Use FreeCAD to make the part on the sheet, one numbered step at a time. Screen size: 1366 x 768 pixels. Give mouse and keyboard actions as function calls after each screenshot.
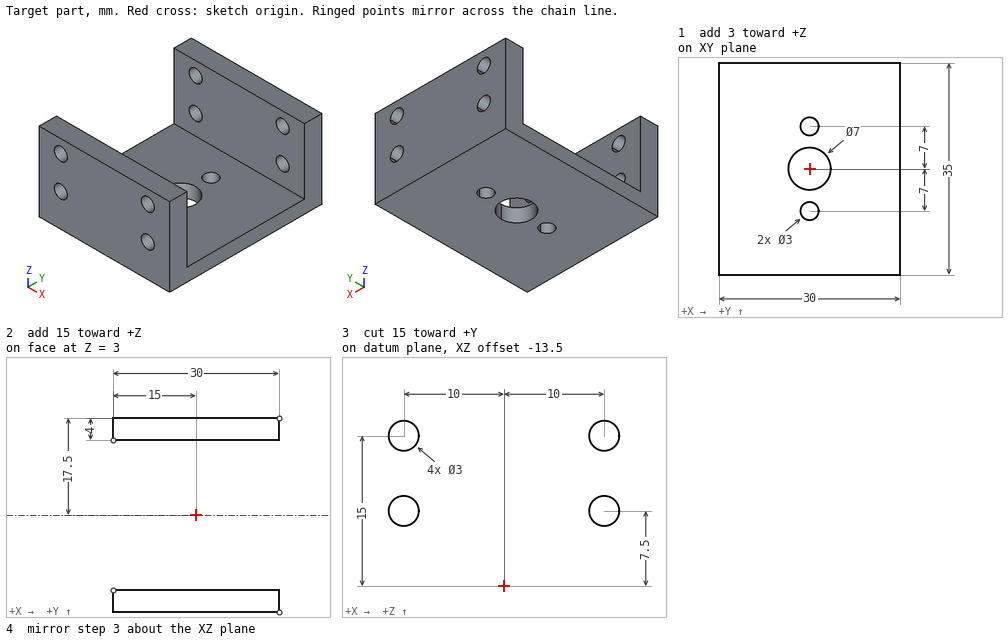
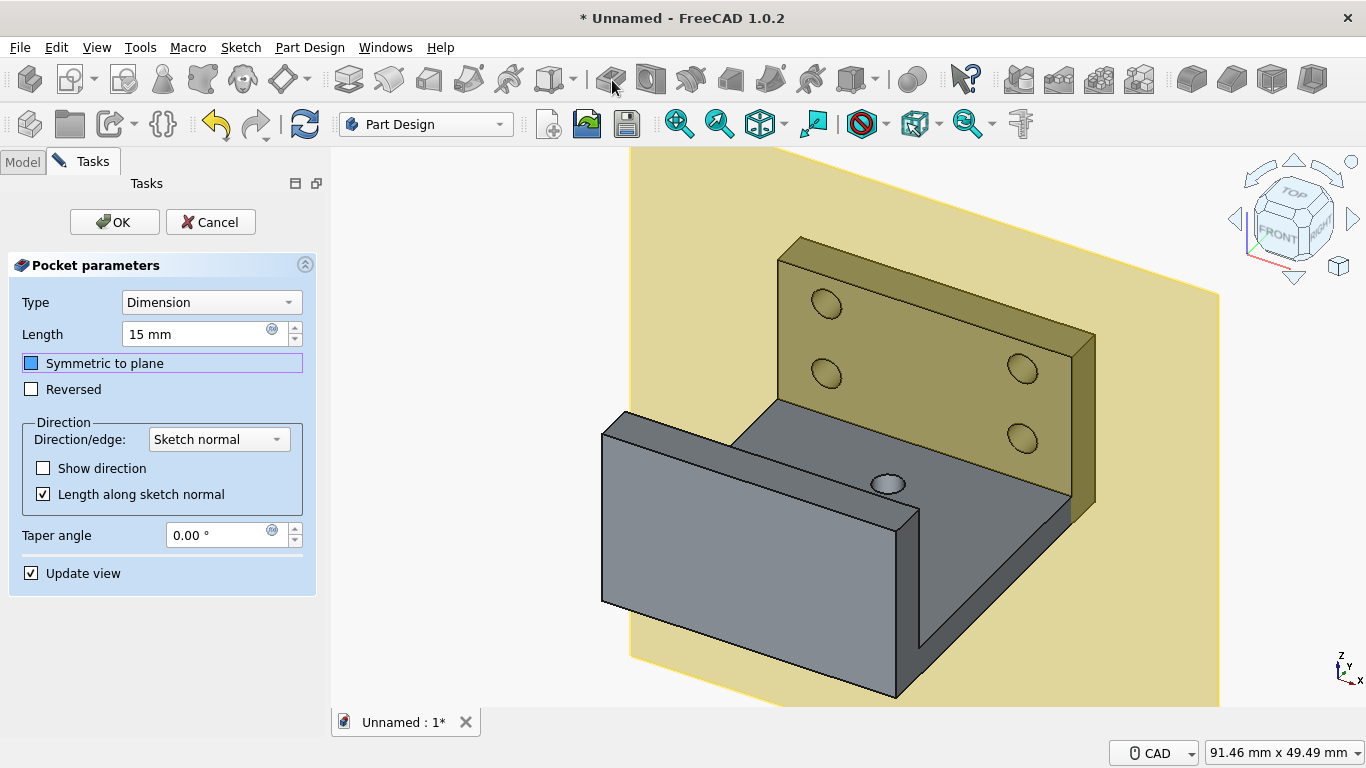
click(115, 222)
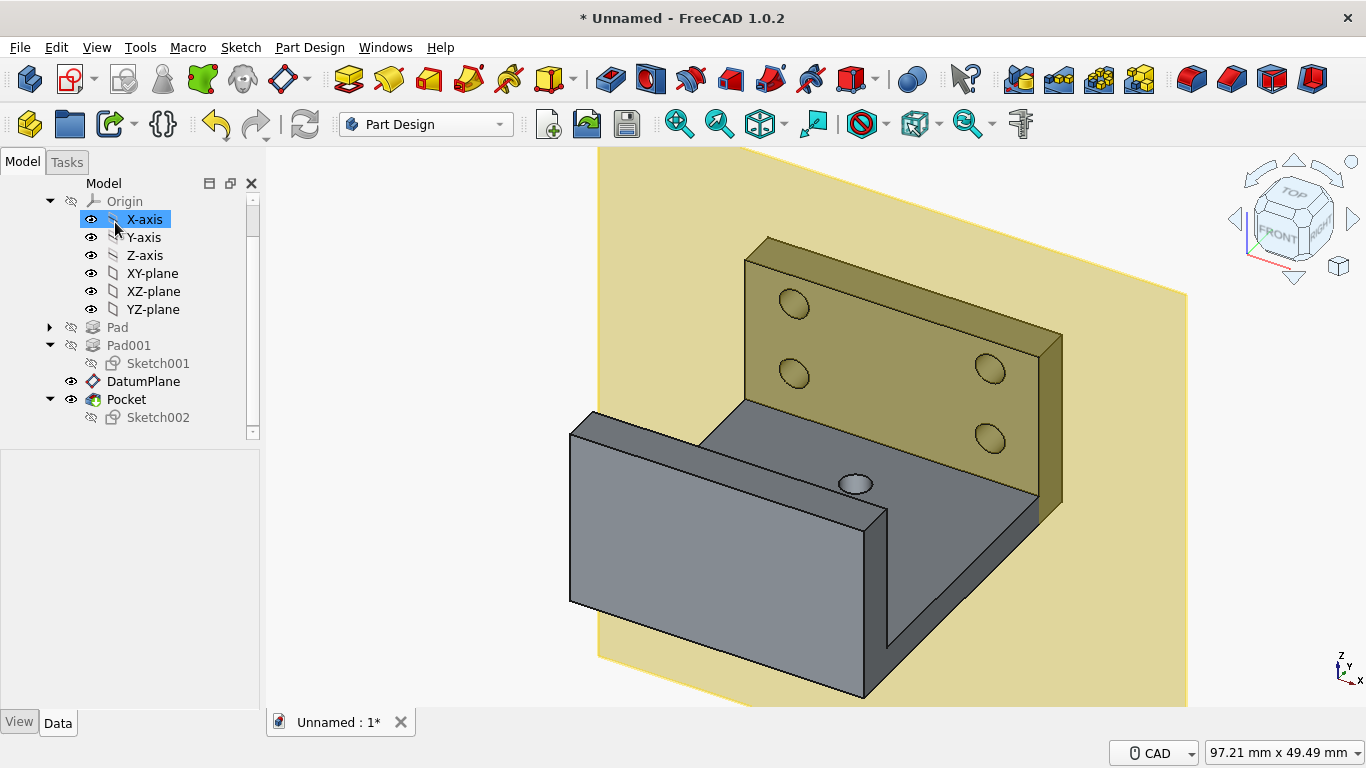
click(116, 381)
key(space)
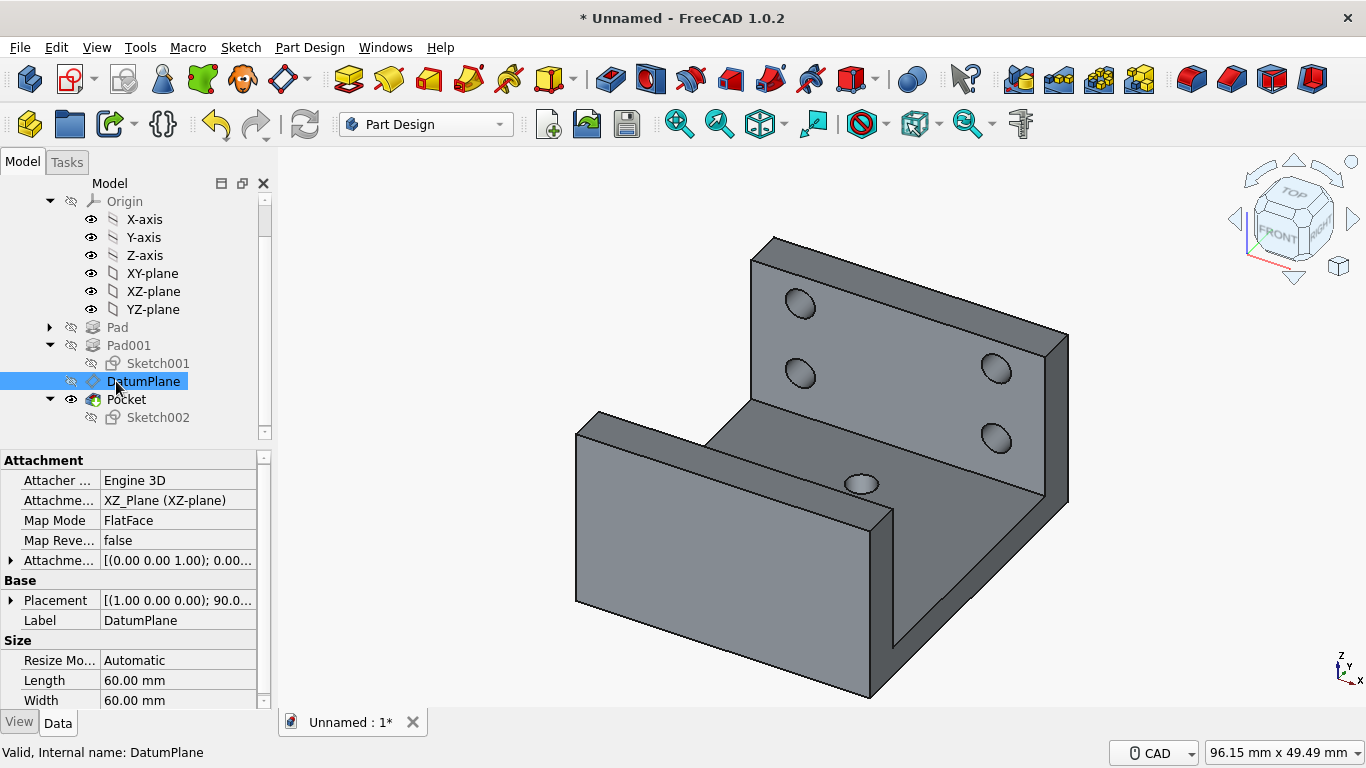
click(116, 399)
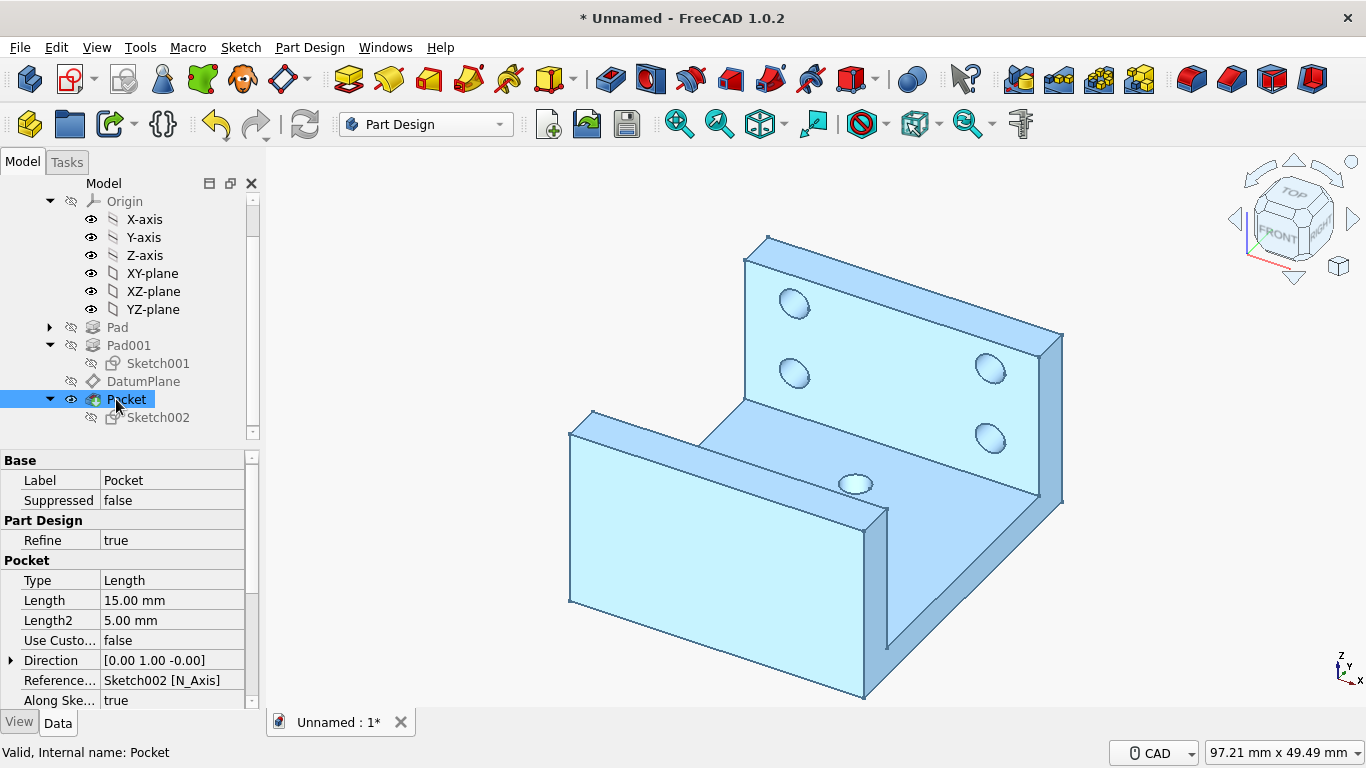
click(1020, 80)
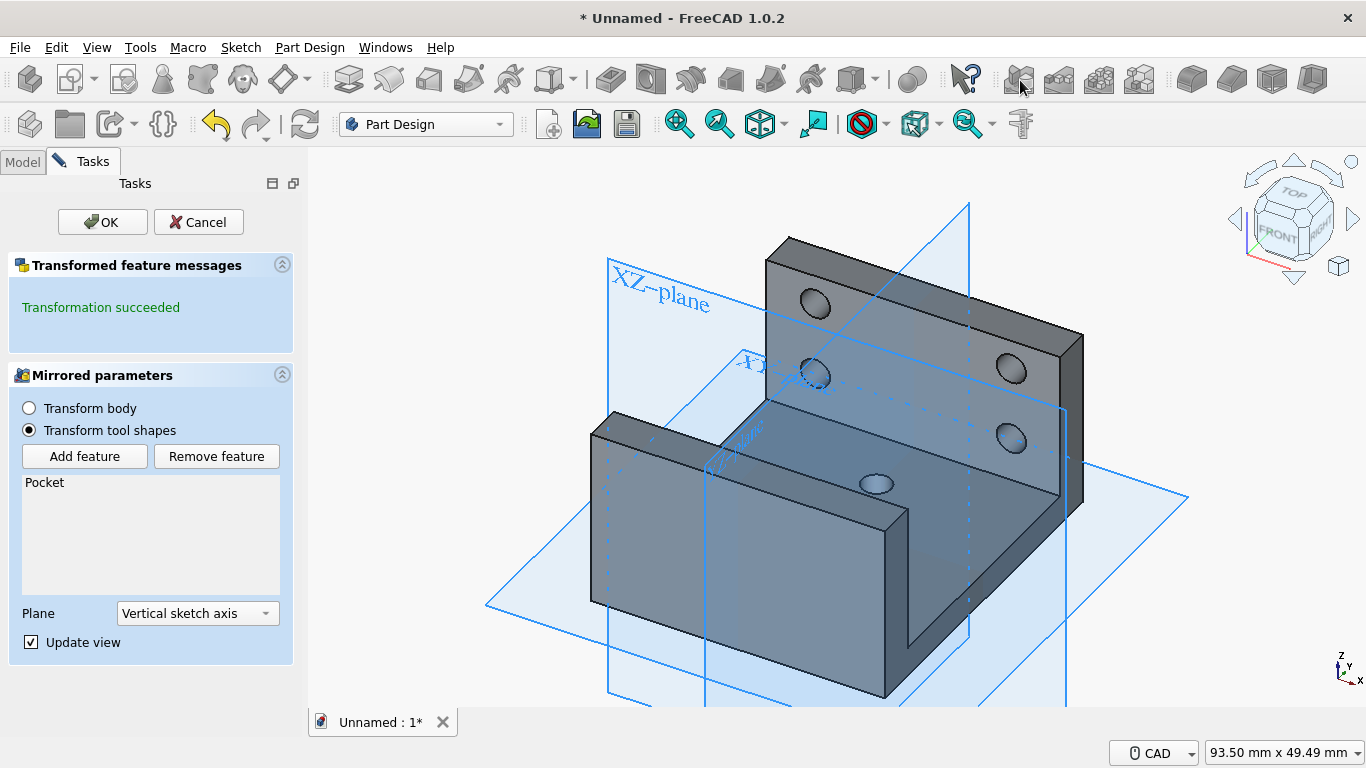
click(198, 614)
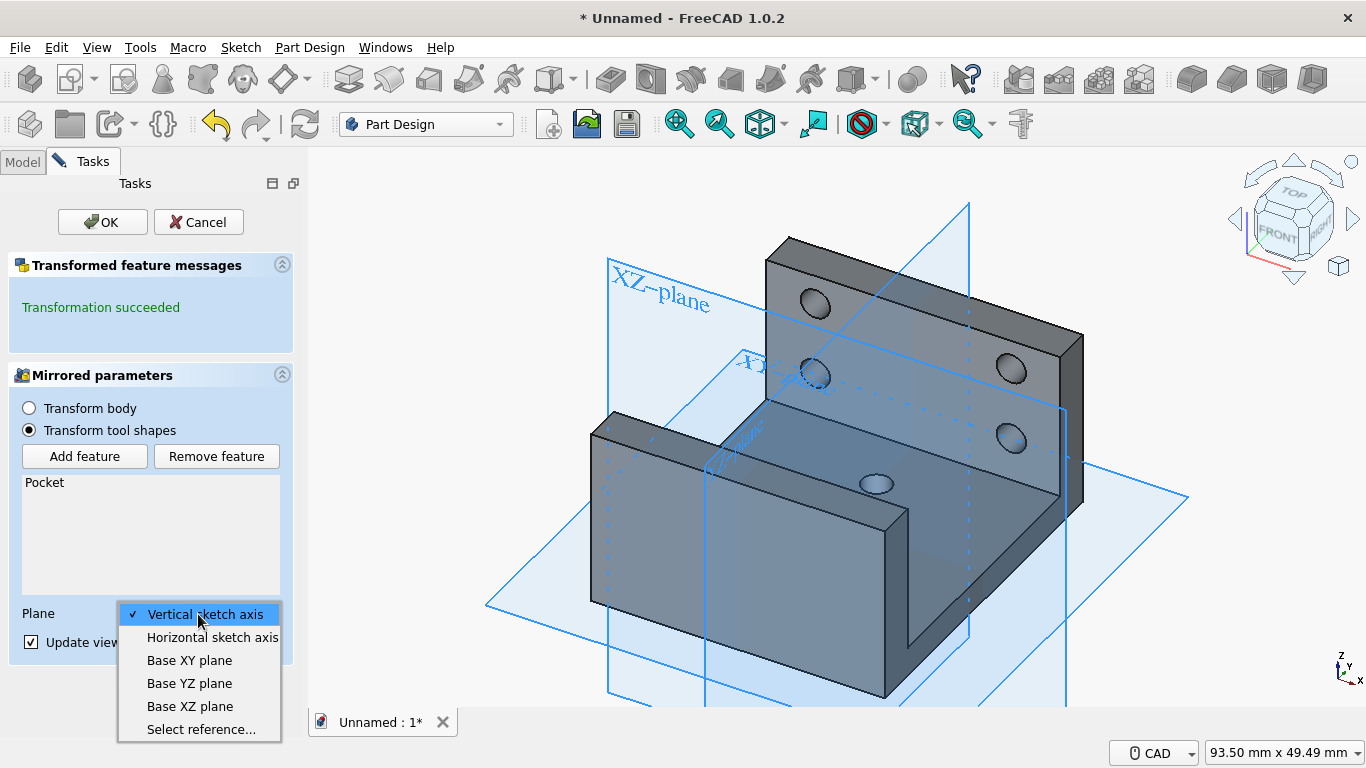
click(198, 706)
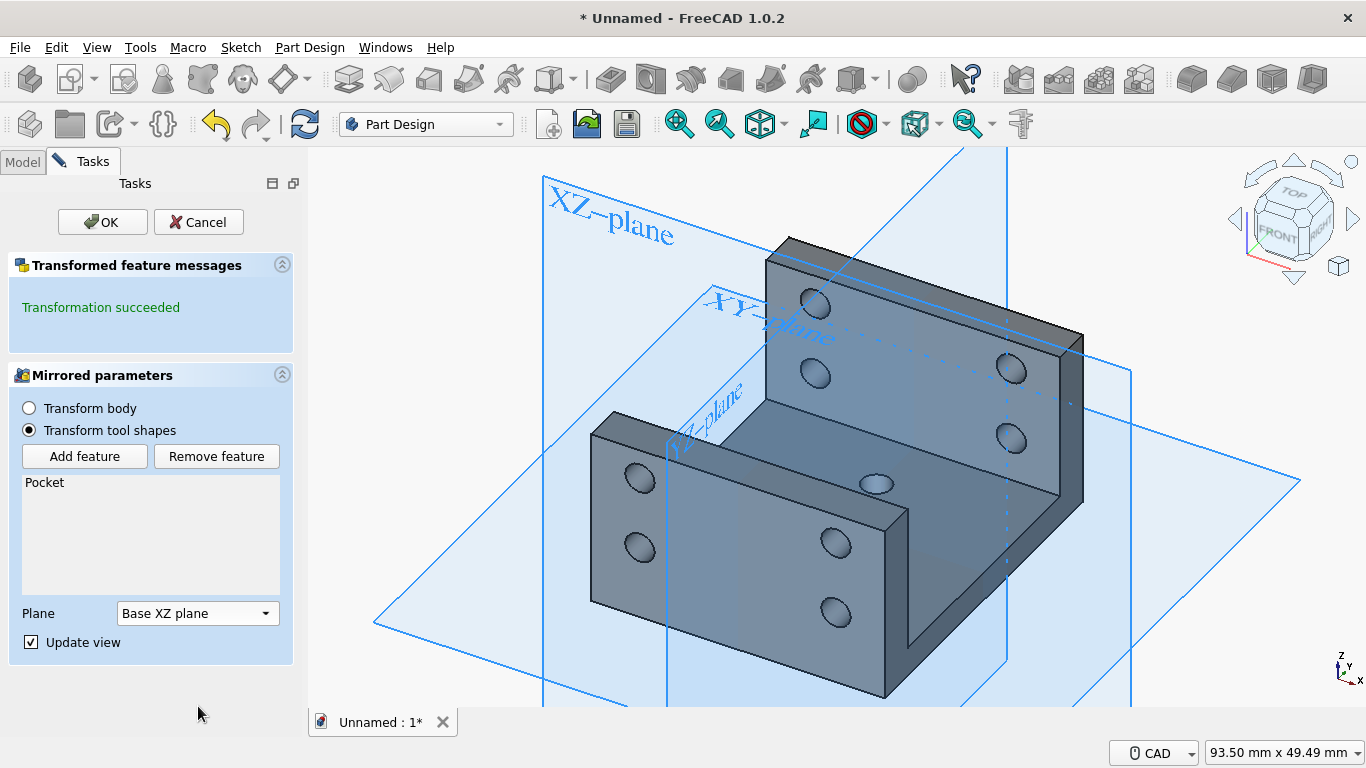
click(103, 222)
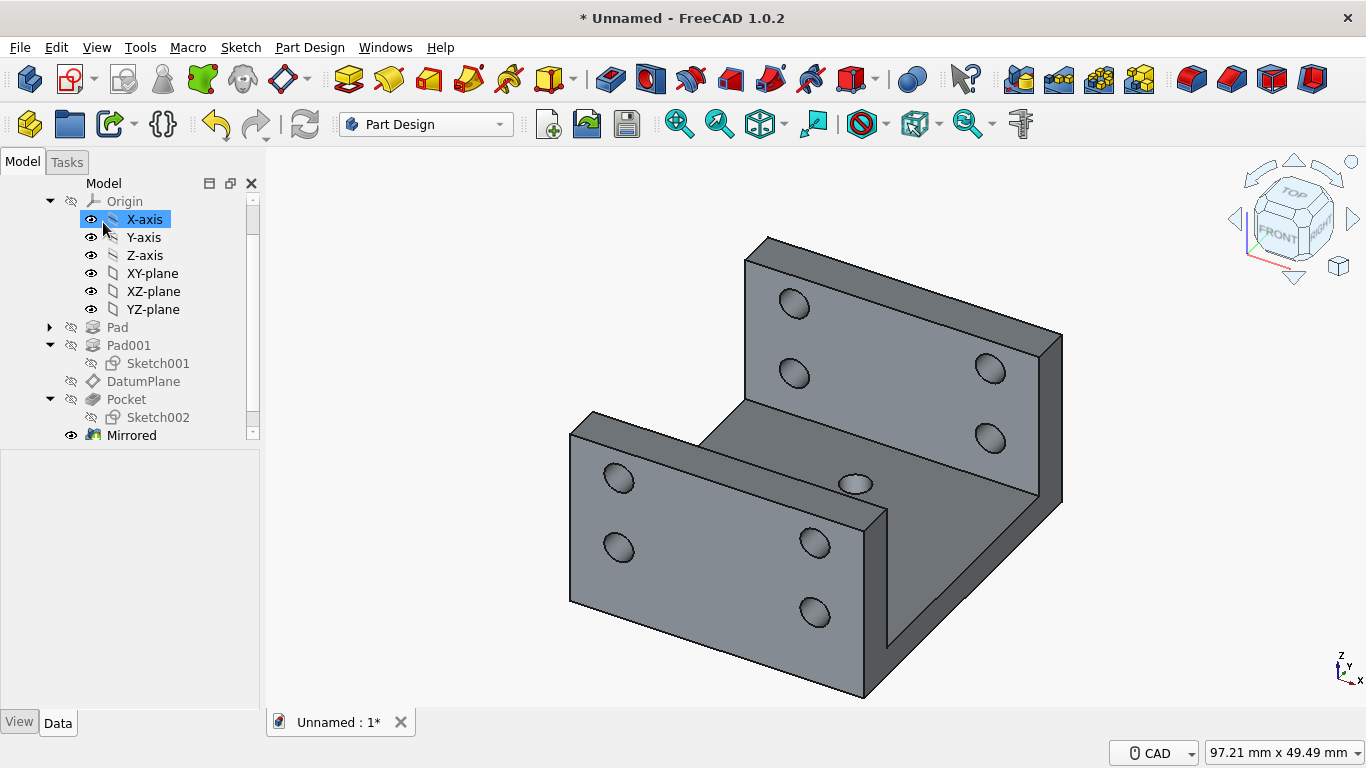
key(0)